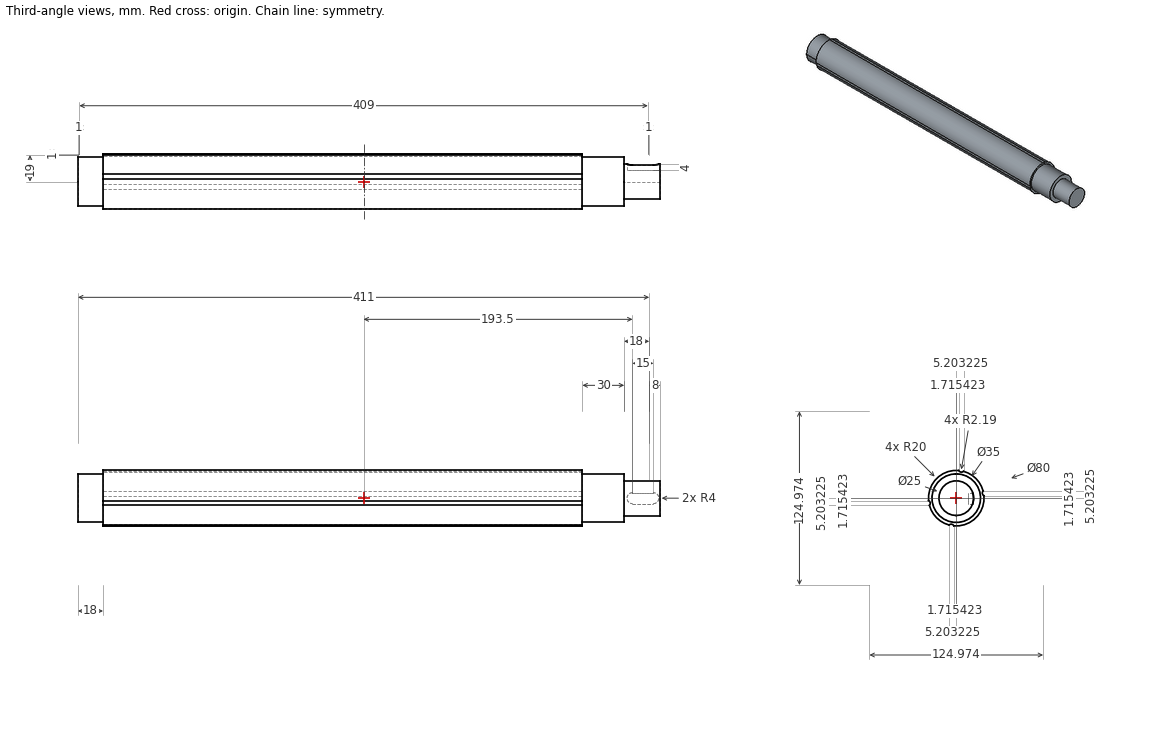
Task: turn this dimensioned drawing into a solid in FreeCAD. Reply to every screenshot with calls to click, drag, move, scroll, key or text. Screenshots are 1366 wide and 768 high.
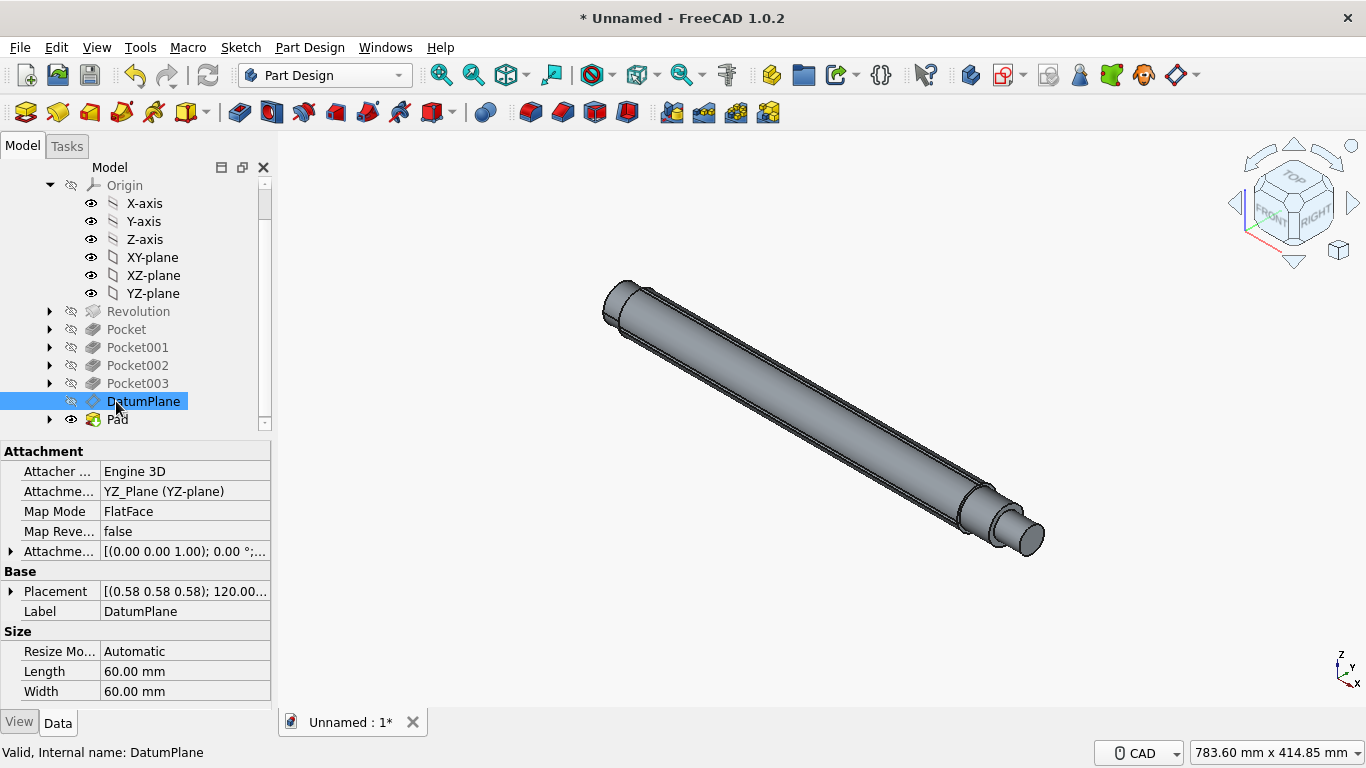
click(136, 275)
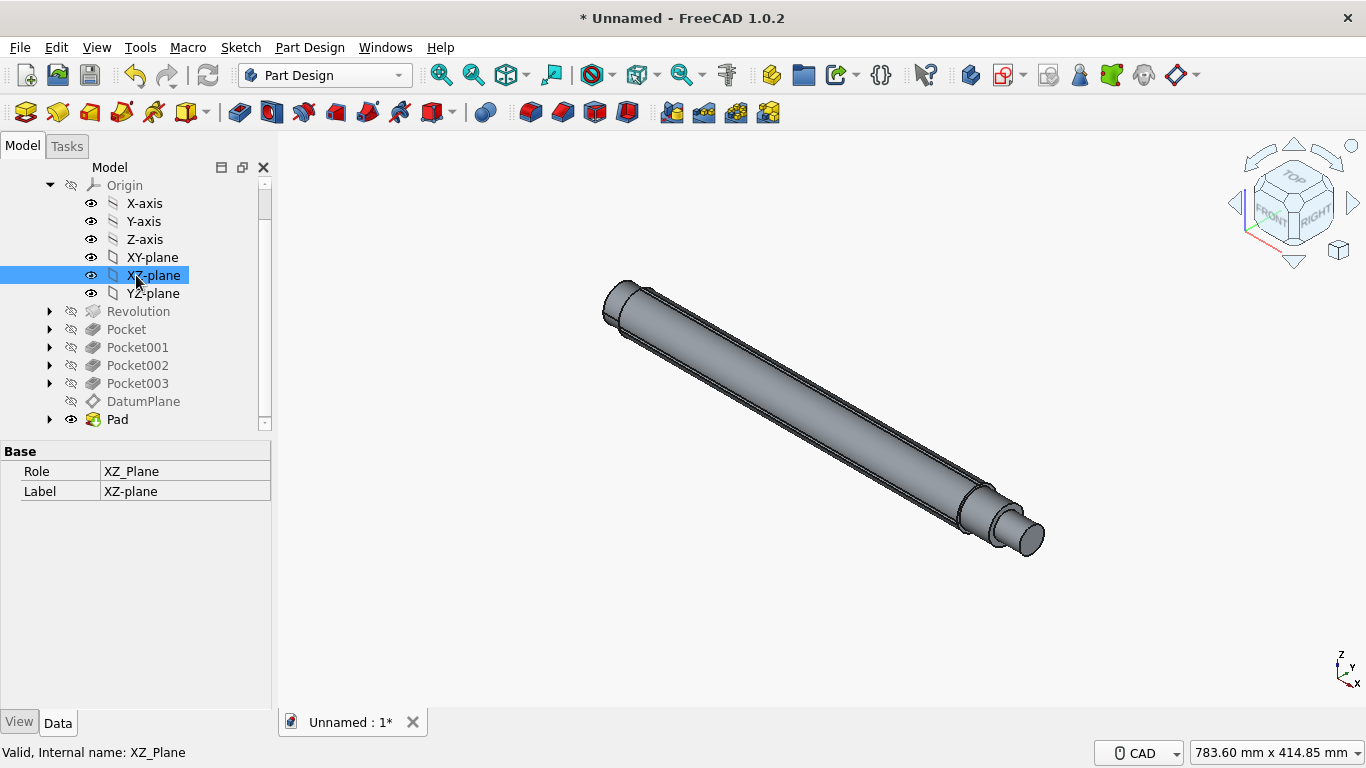
click(1176, 76)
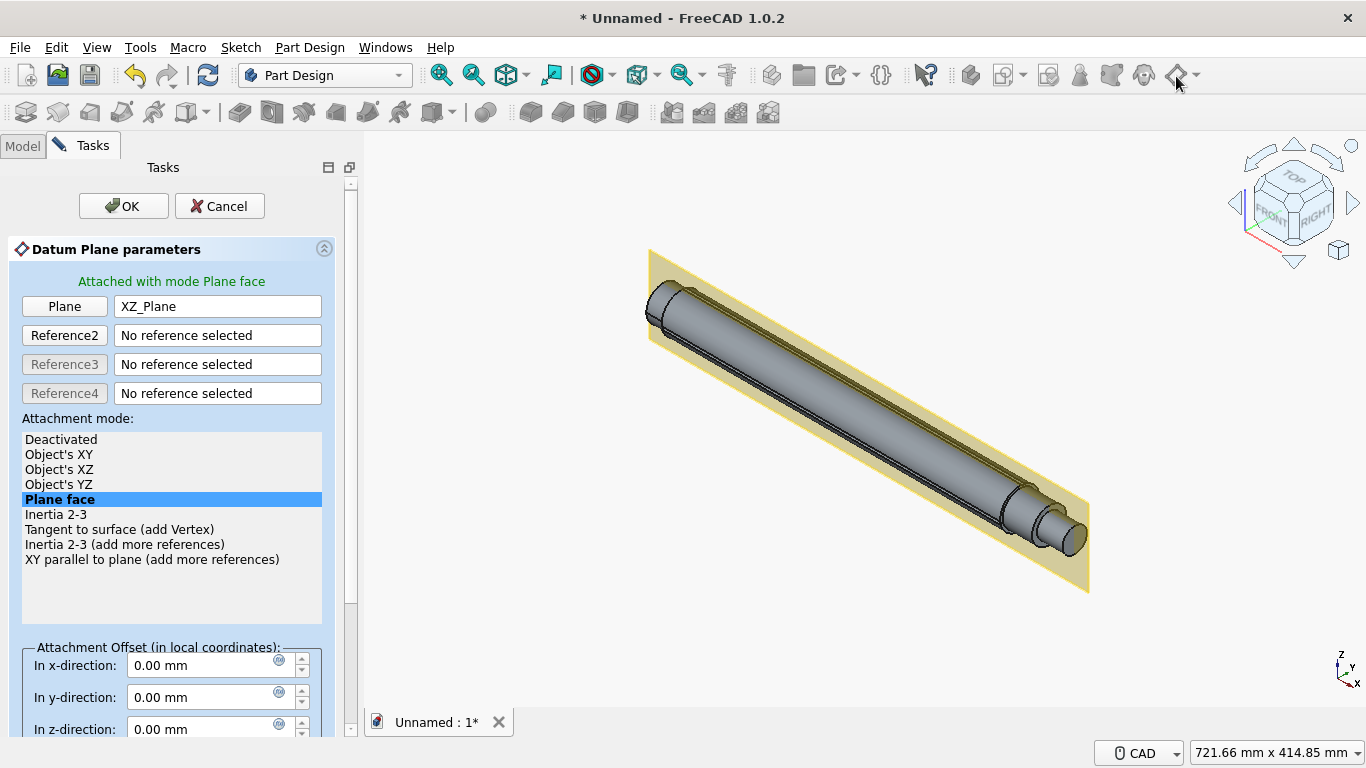
scroll(351, 456, down, 2)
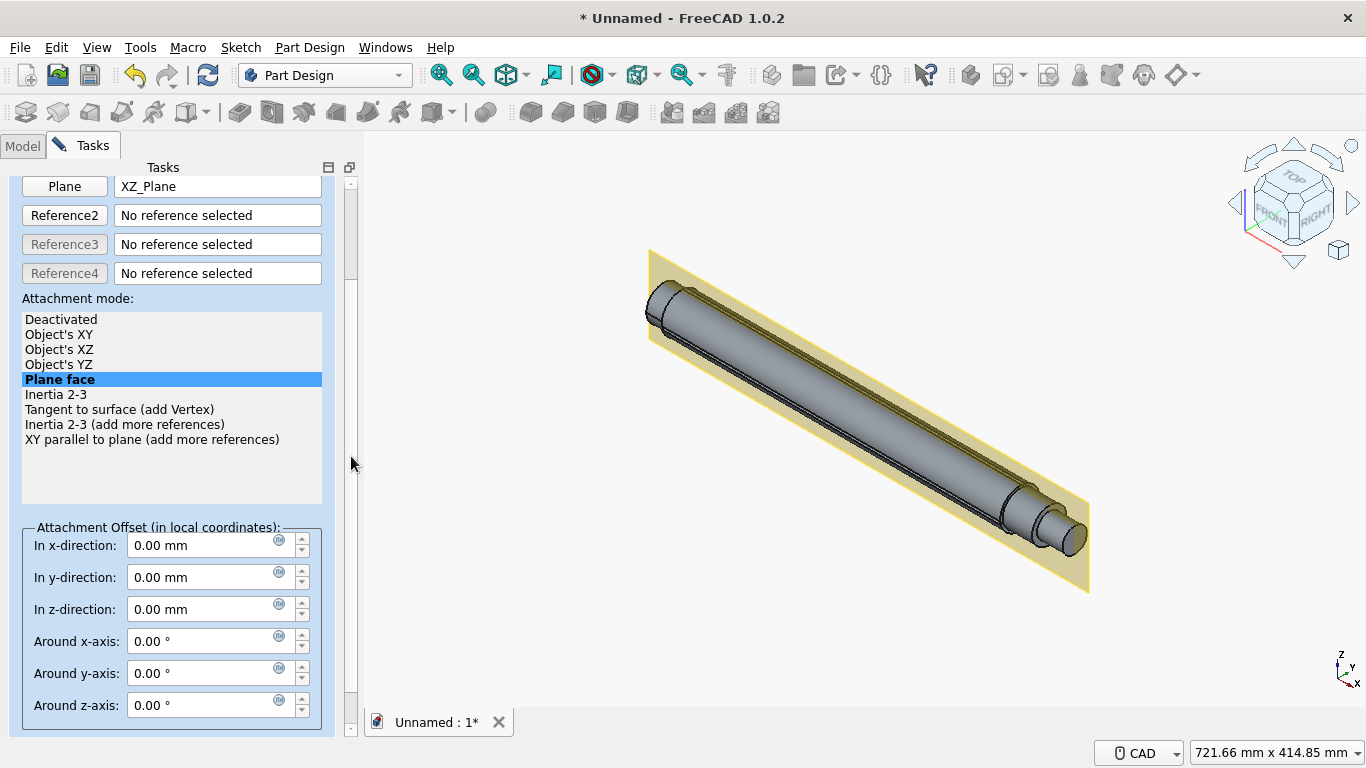
triple_click(210, 609)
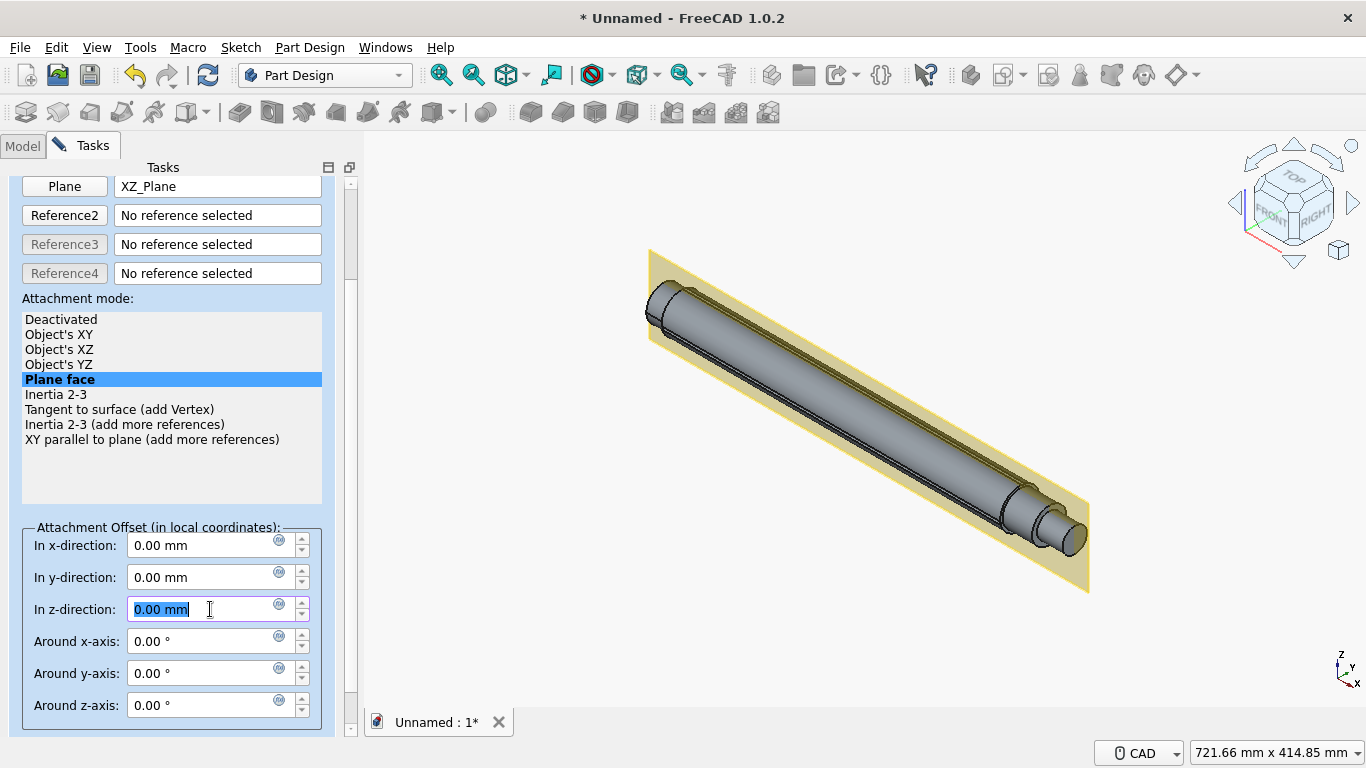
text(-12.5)
key(Tab)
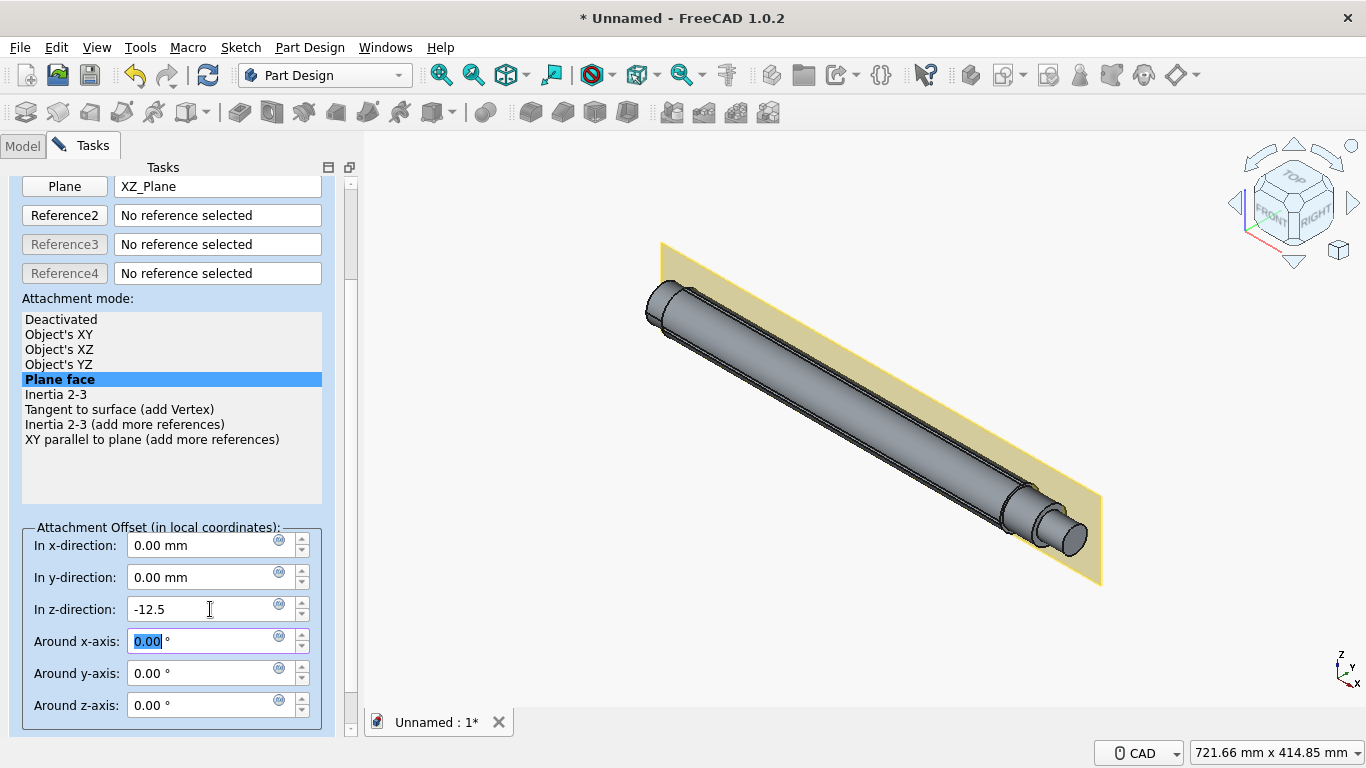
scroll(351, 456, up, 3)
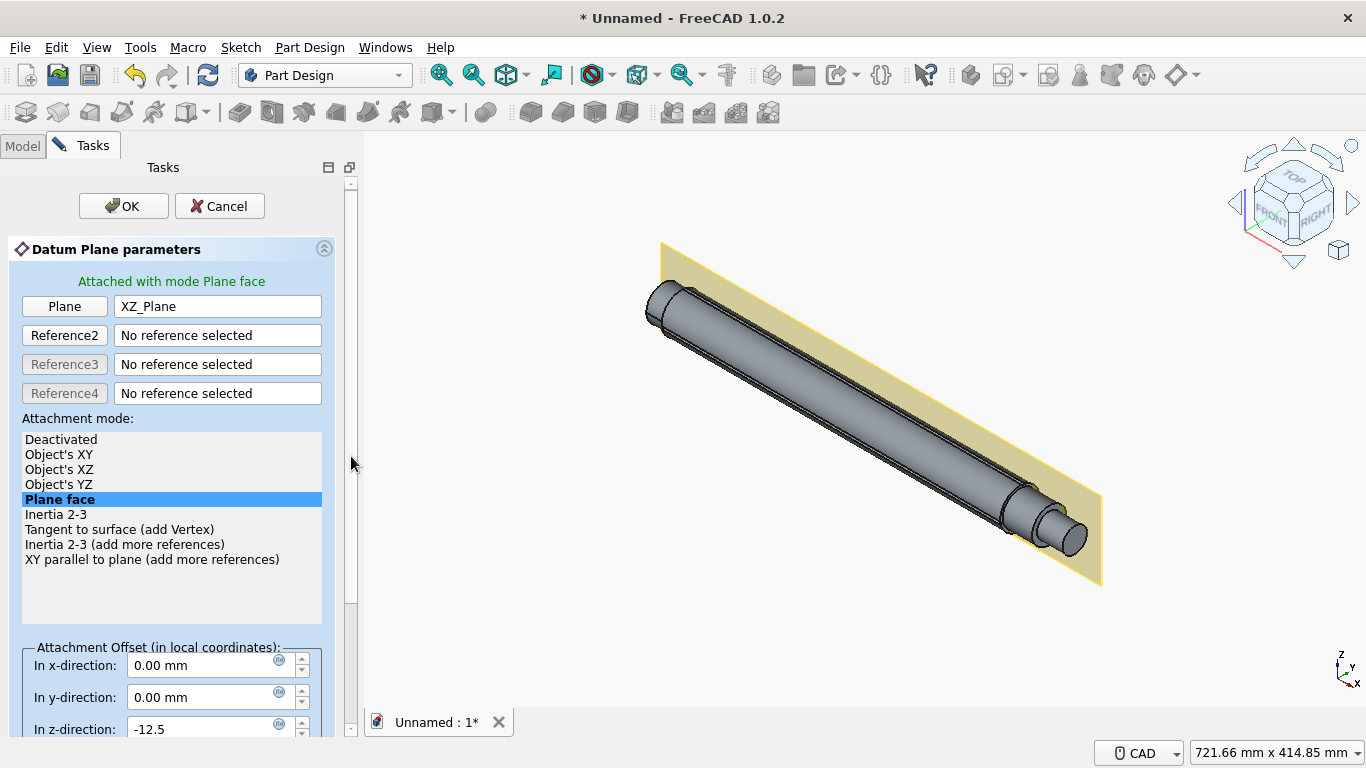
click(124, 206)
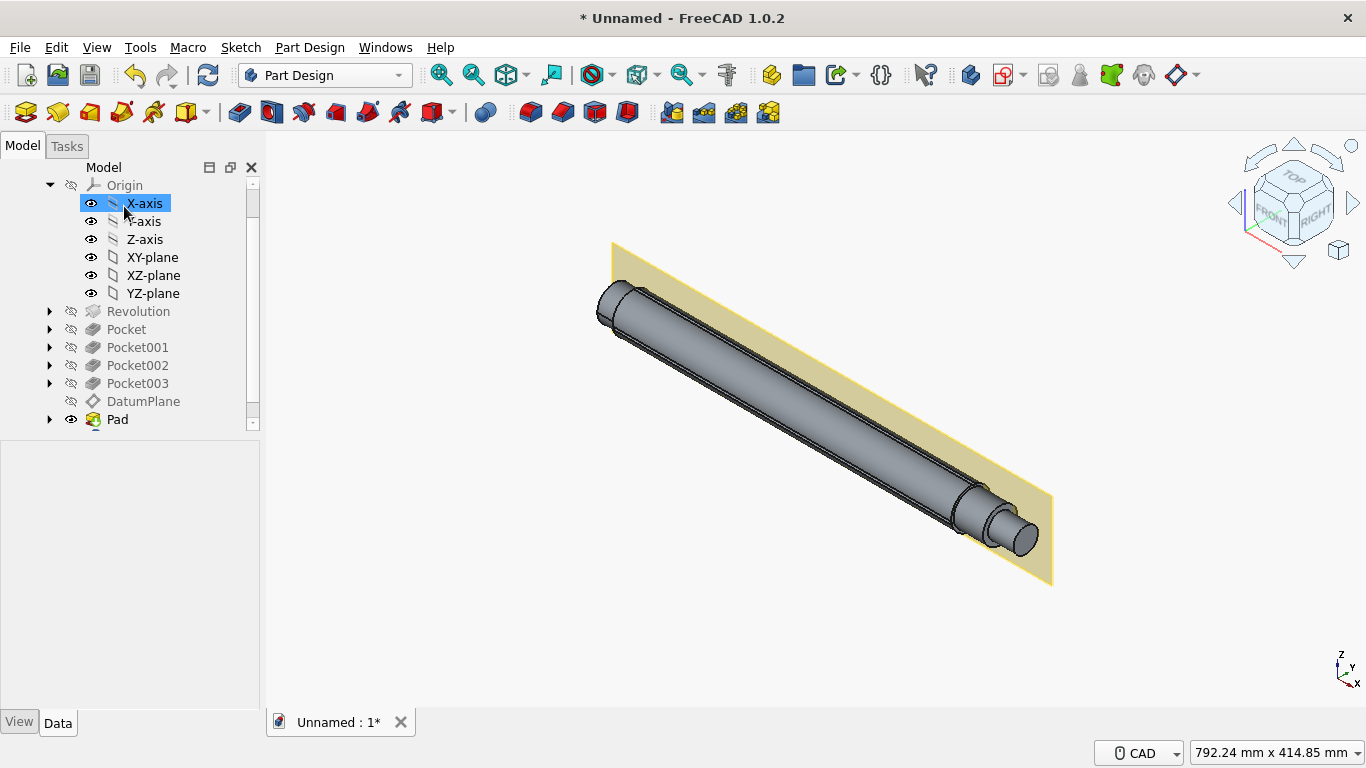
scroll(140, 307, down, 3)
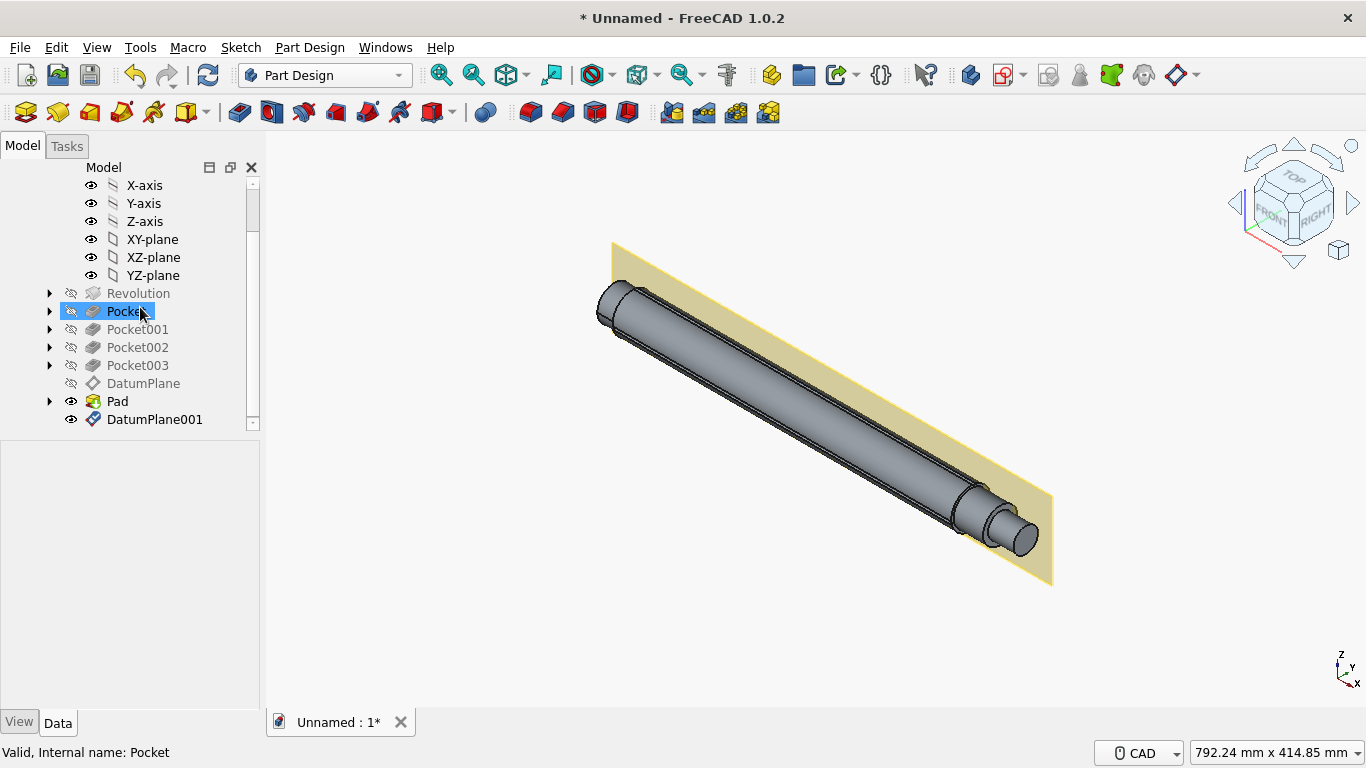
click(116, 419)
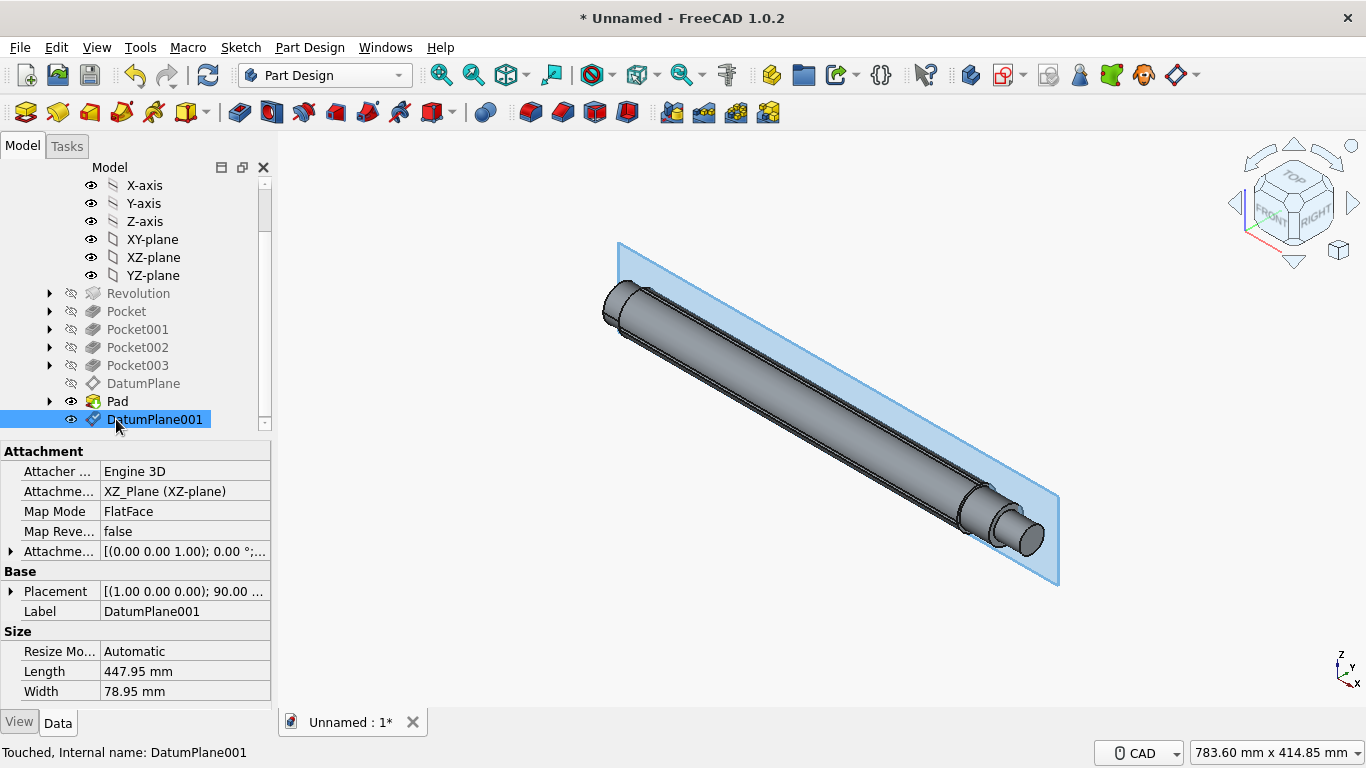
click(1004, 76)